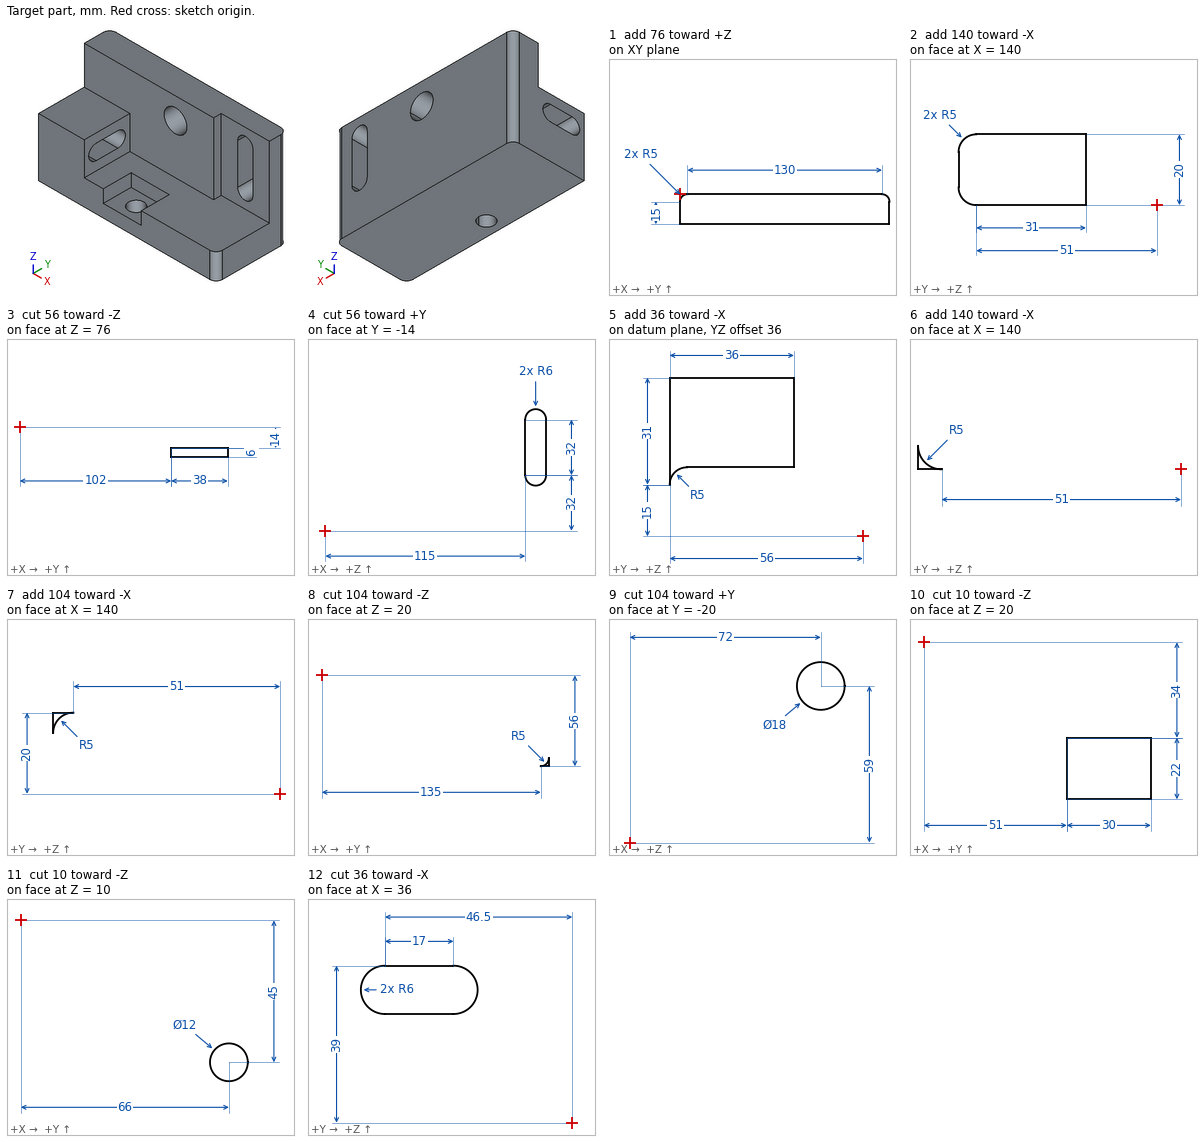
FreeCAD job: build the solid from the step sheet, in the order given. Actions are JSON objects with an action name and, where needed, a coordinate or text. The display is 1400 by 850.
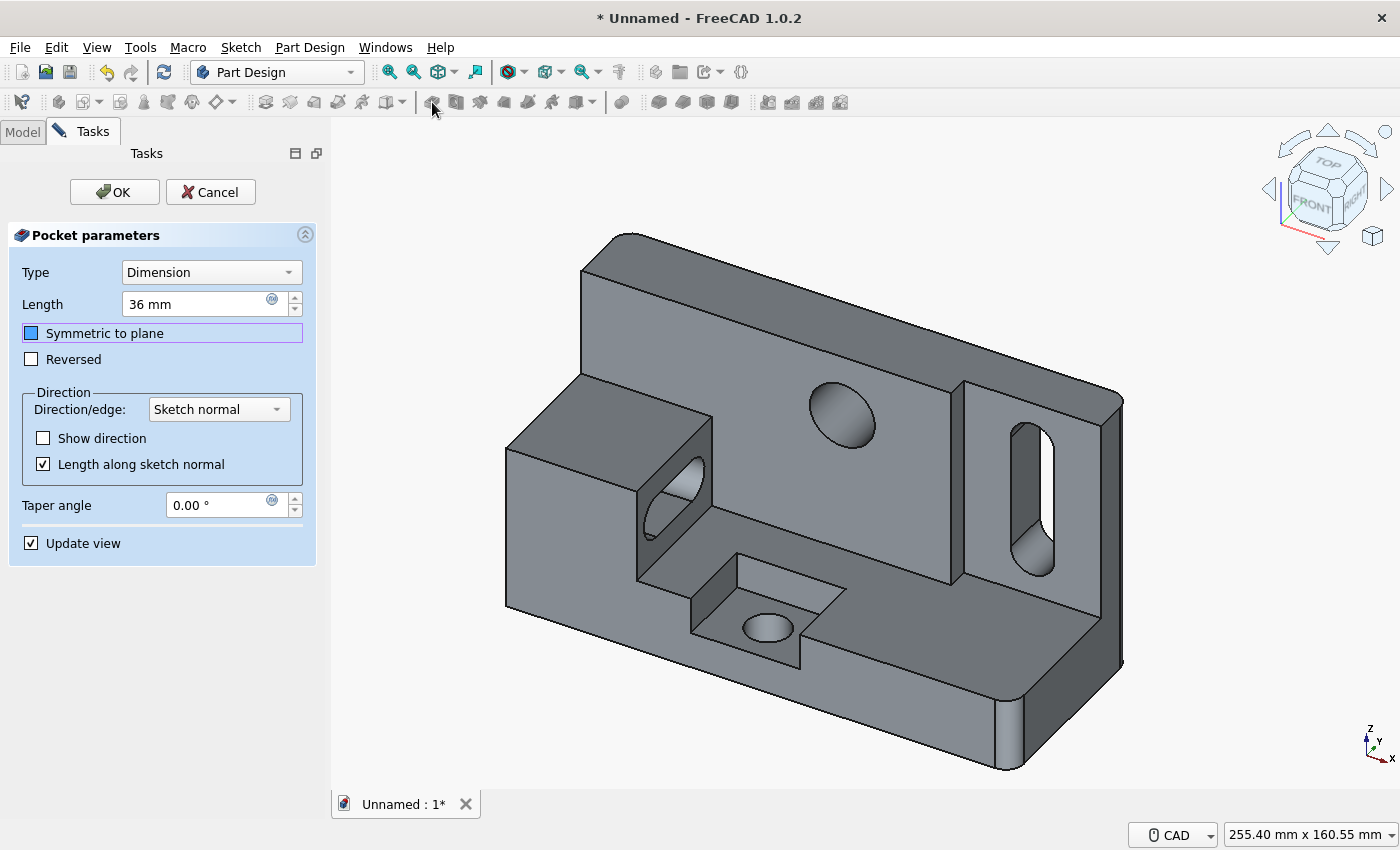
{"action": "left_click", "coordinate": [115, 192]}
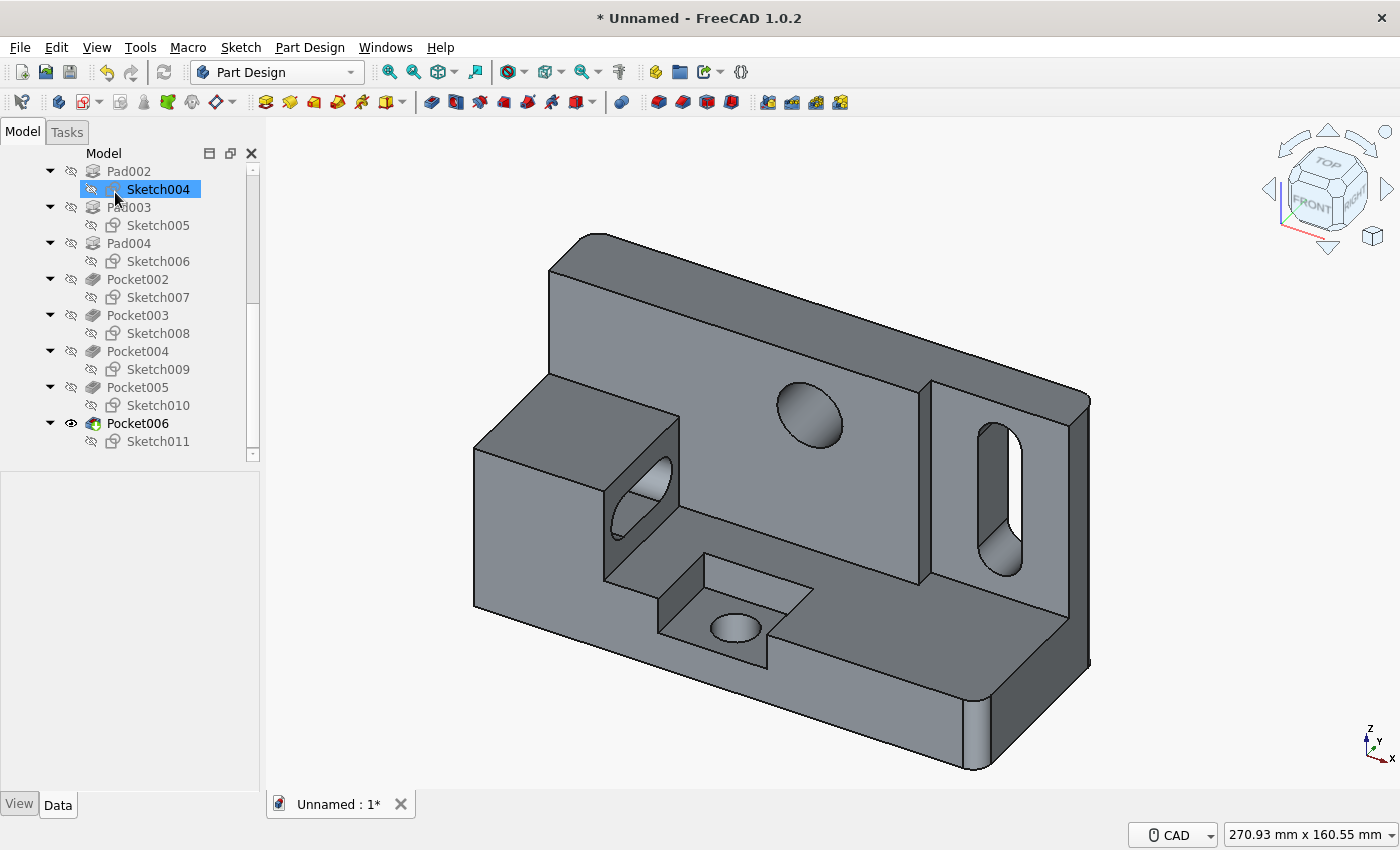
{"action": "key", "text": "0"}